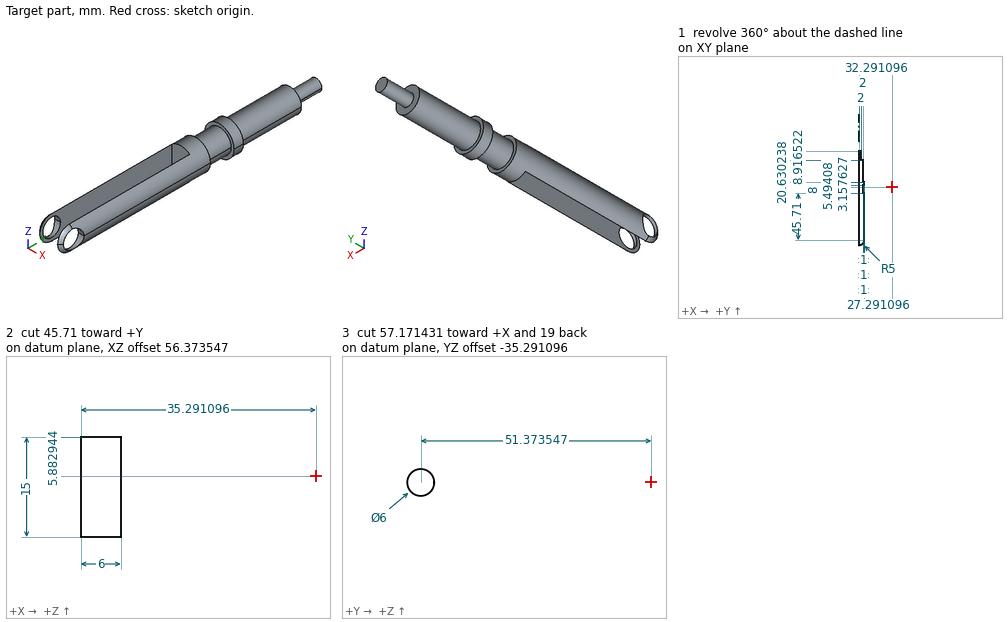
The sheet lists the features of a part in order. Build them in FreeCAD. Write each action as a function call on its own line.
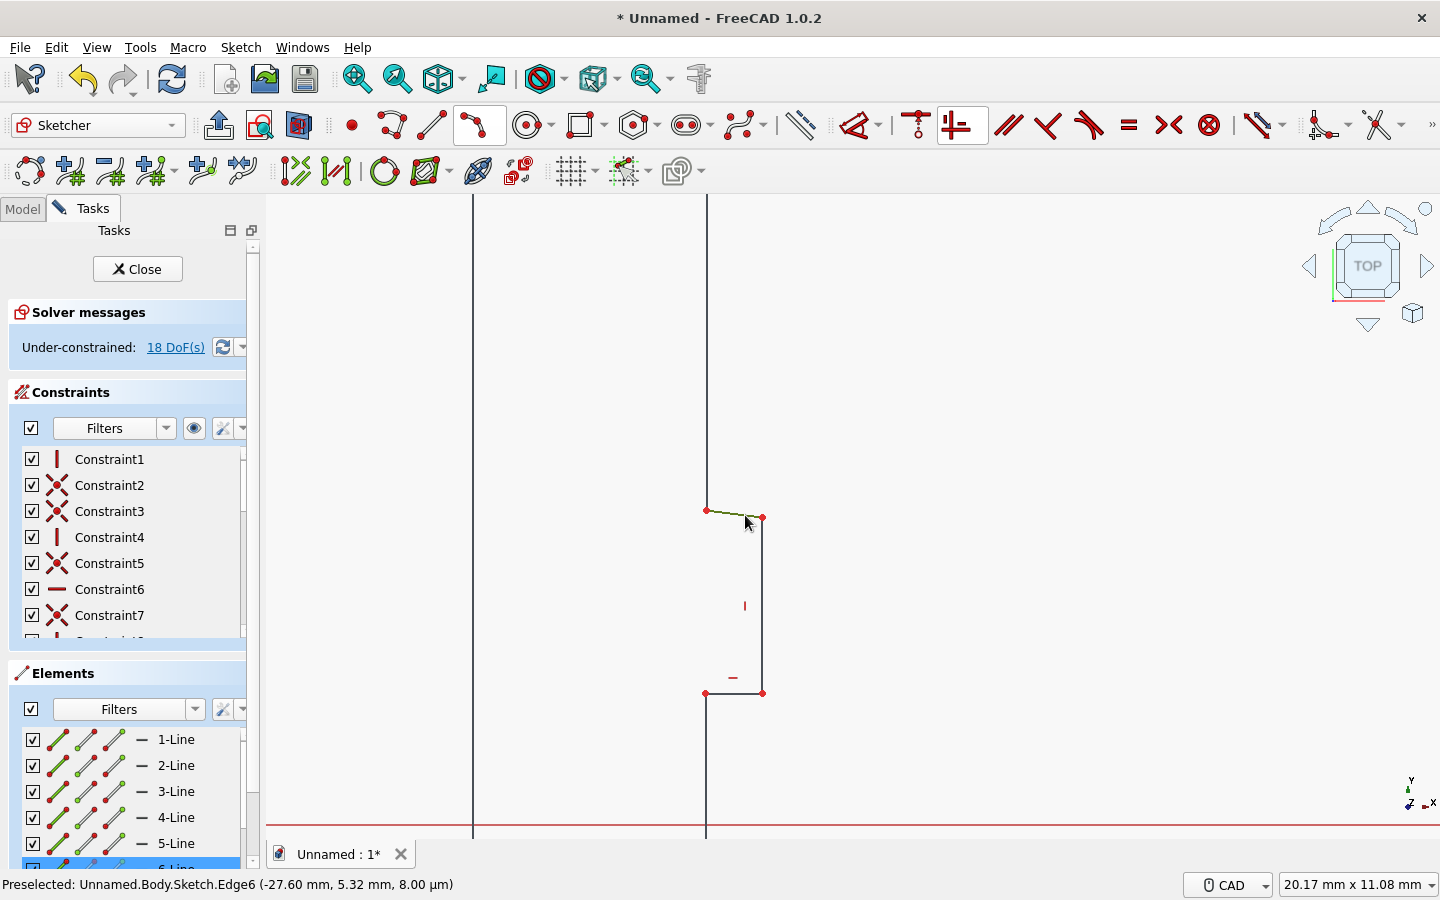
click(982, 126)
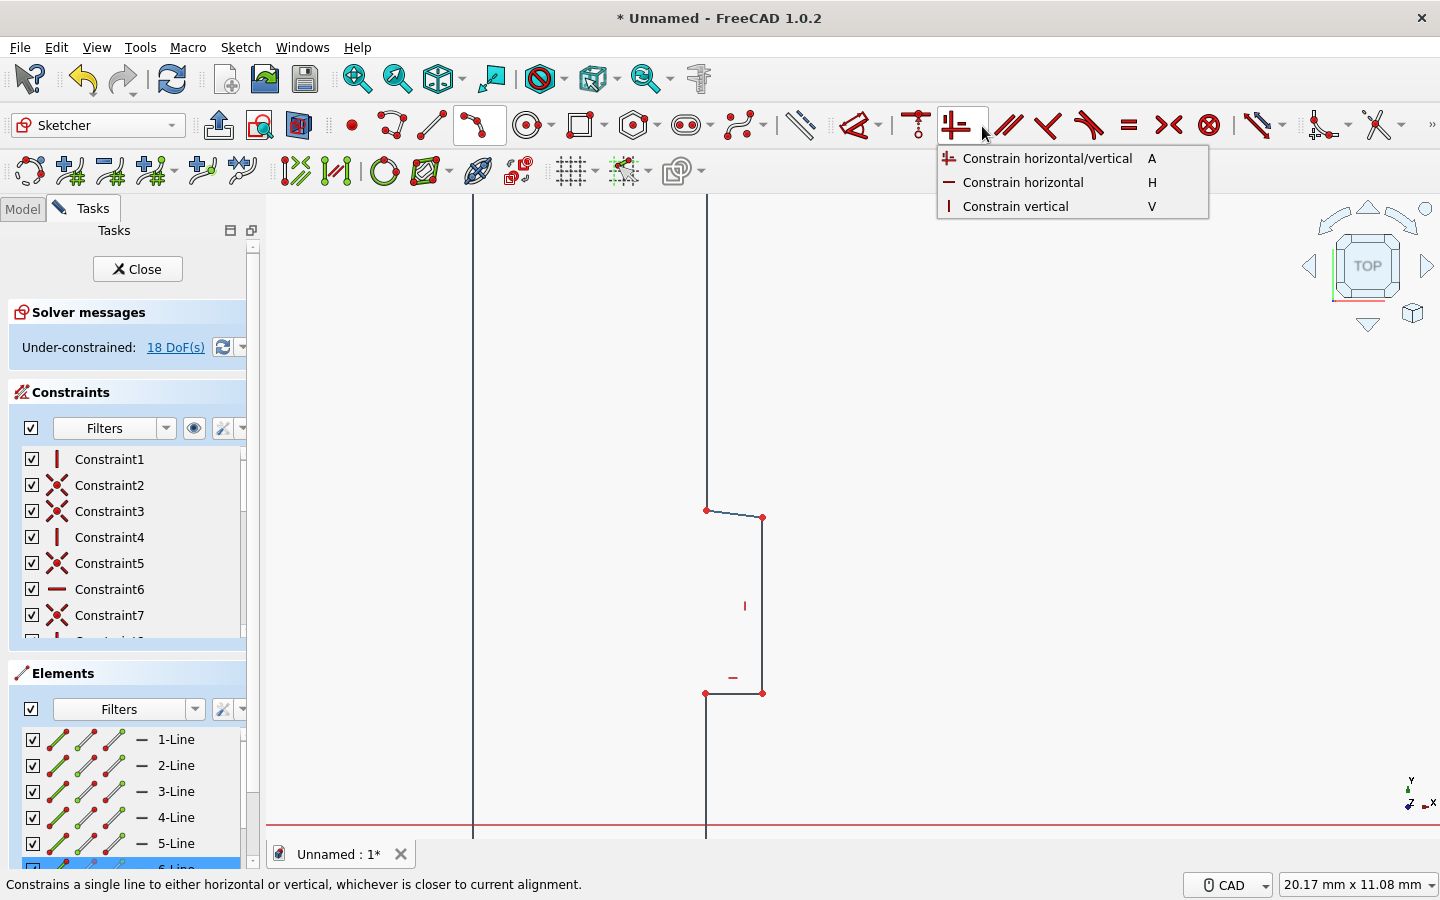
click(1073, 182)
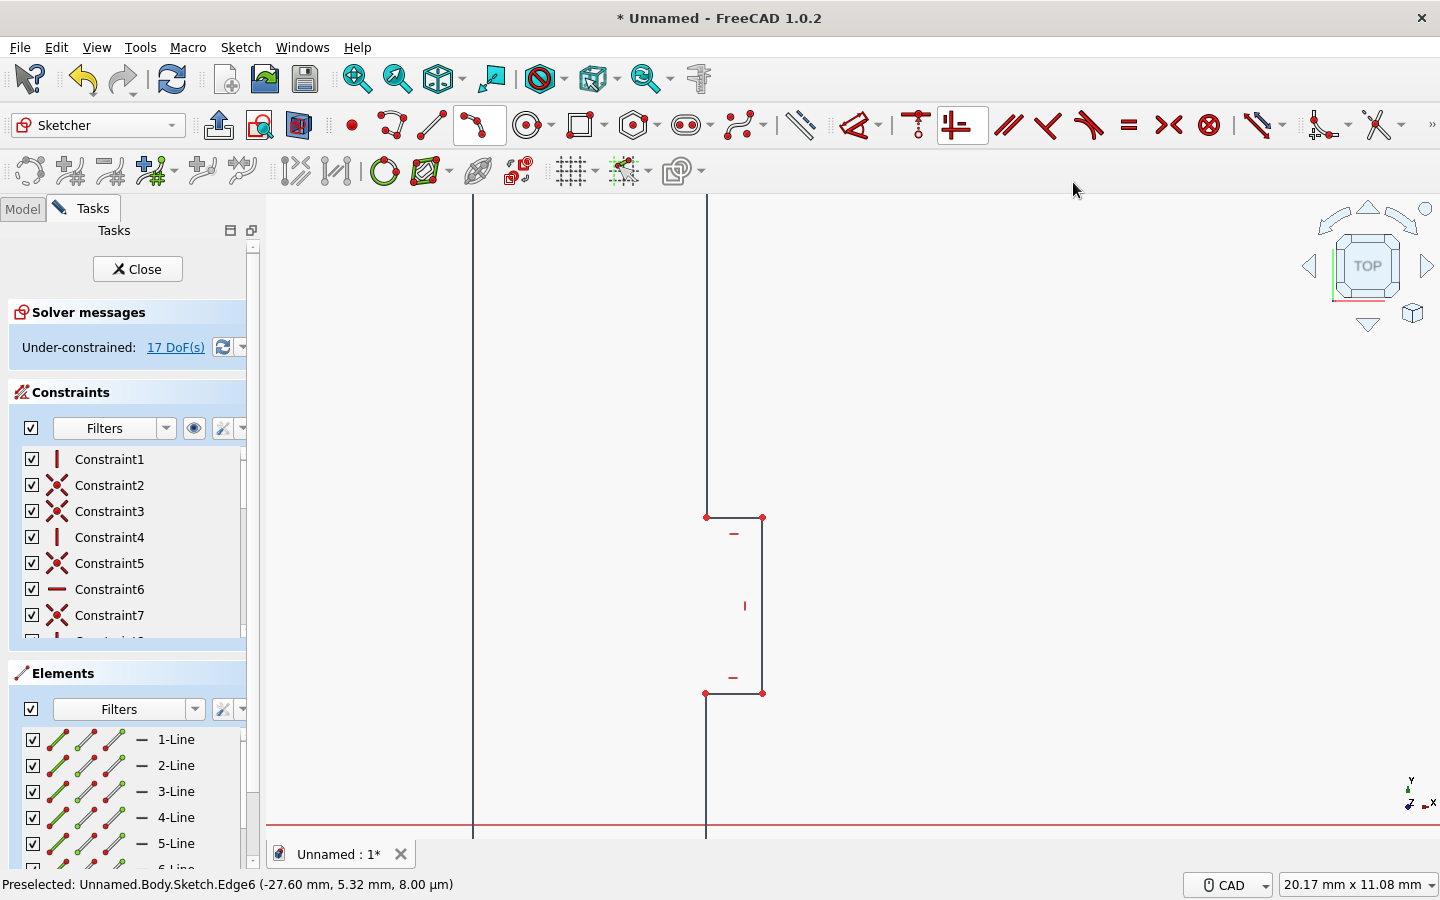
scroll(744, 525, down, 14)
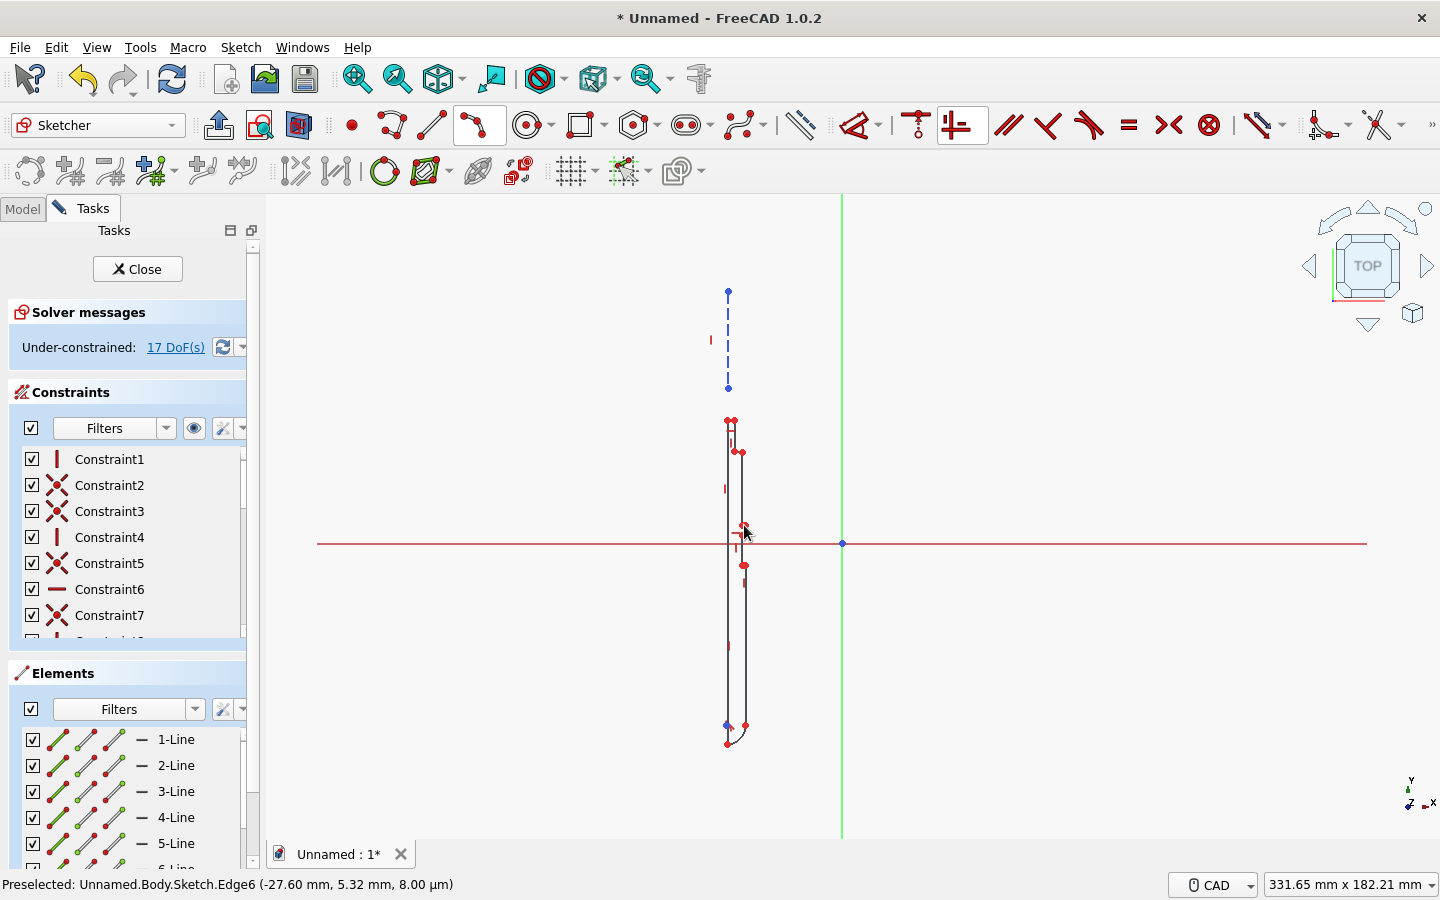
scroll(740, 452, up, 10)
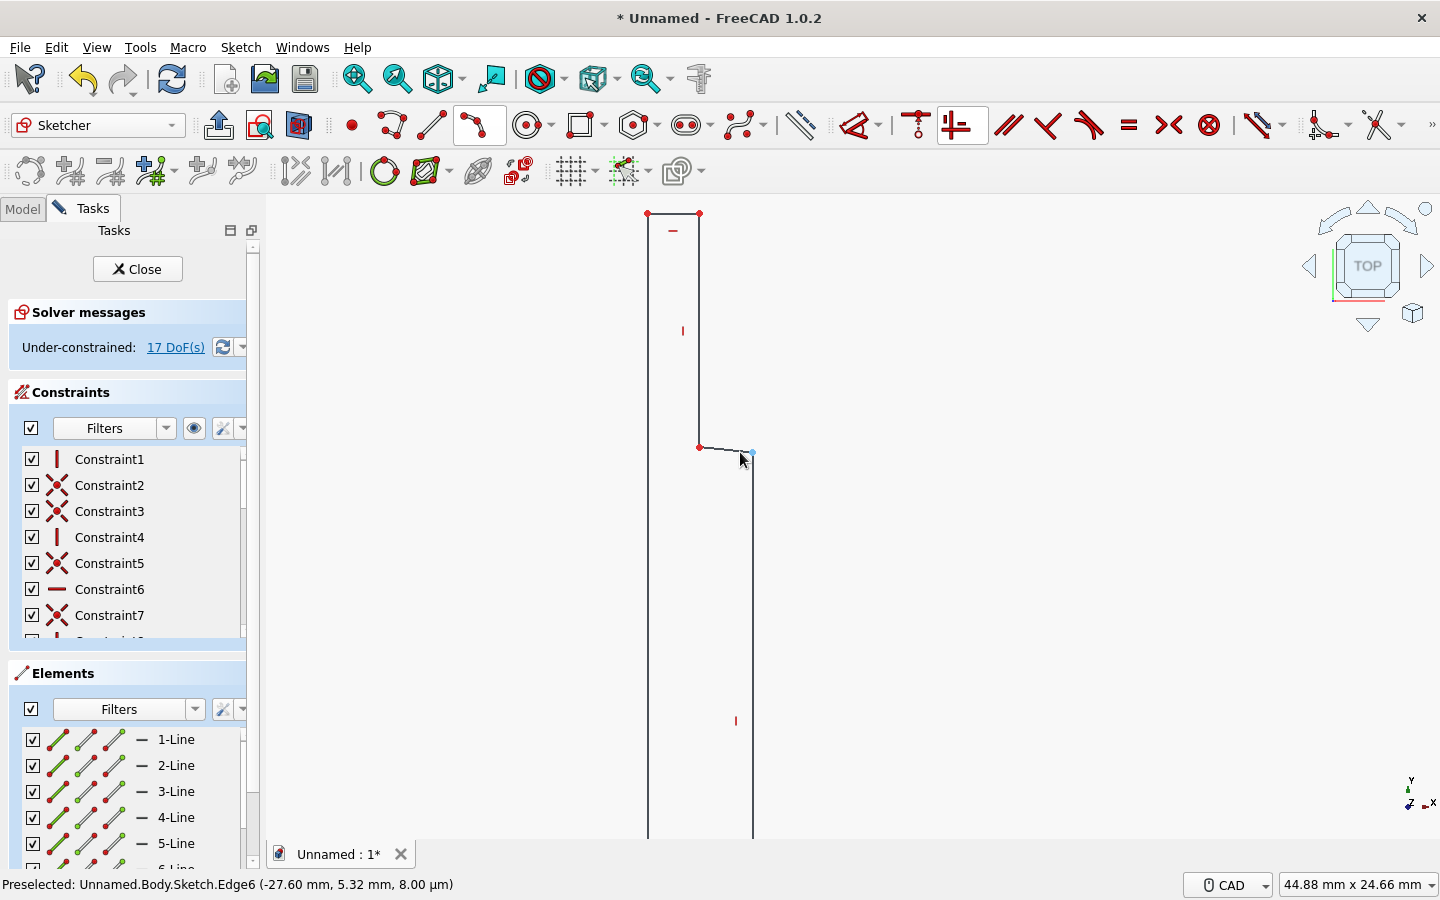
click(737, 451)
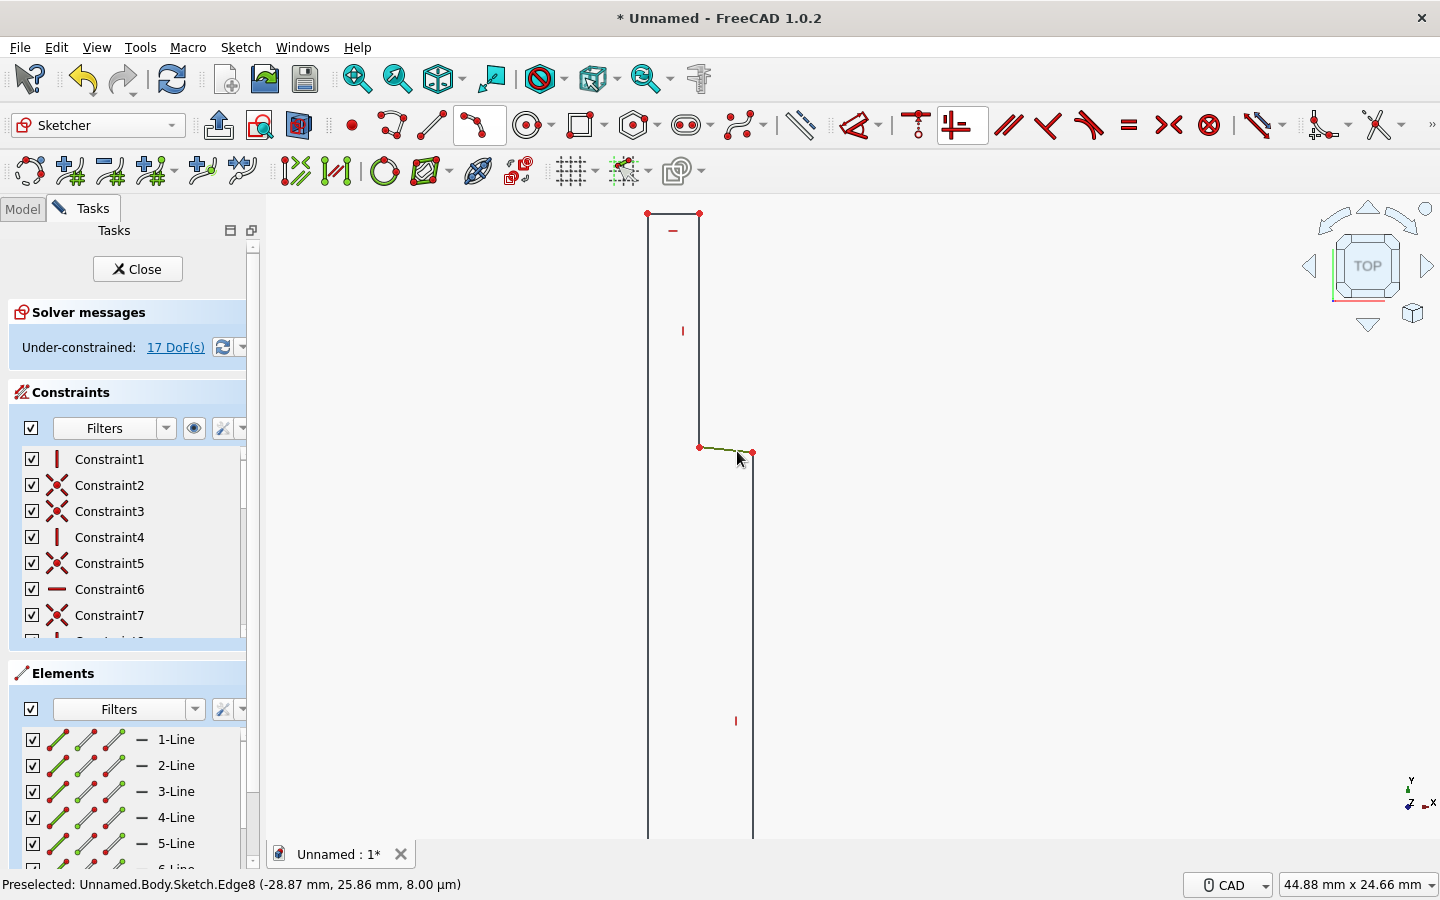
key(h)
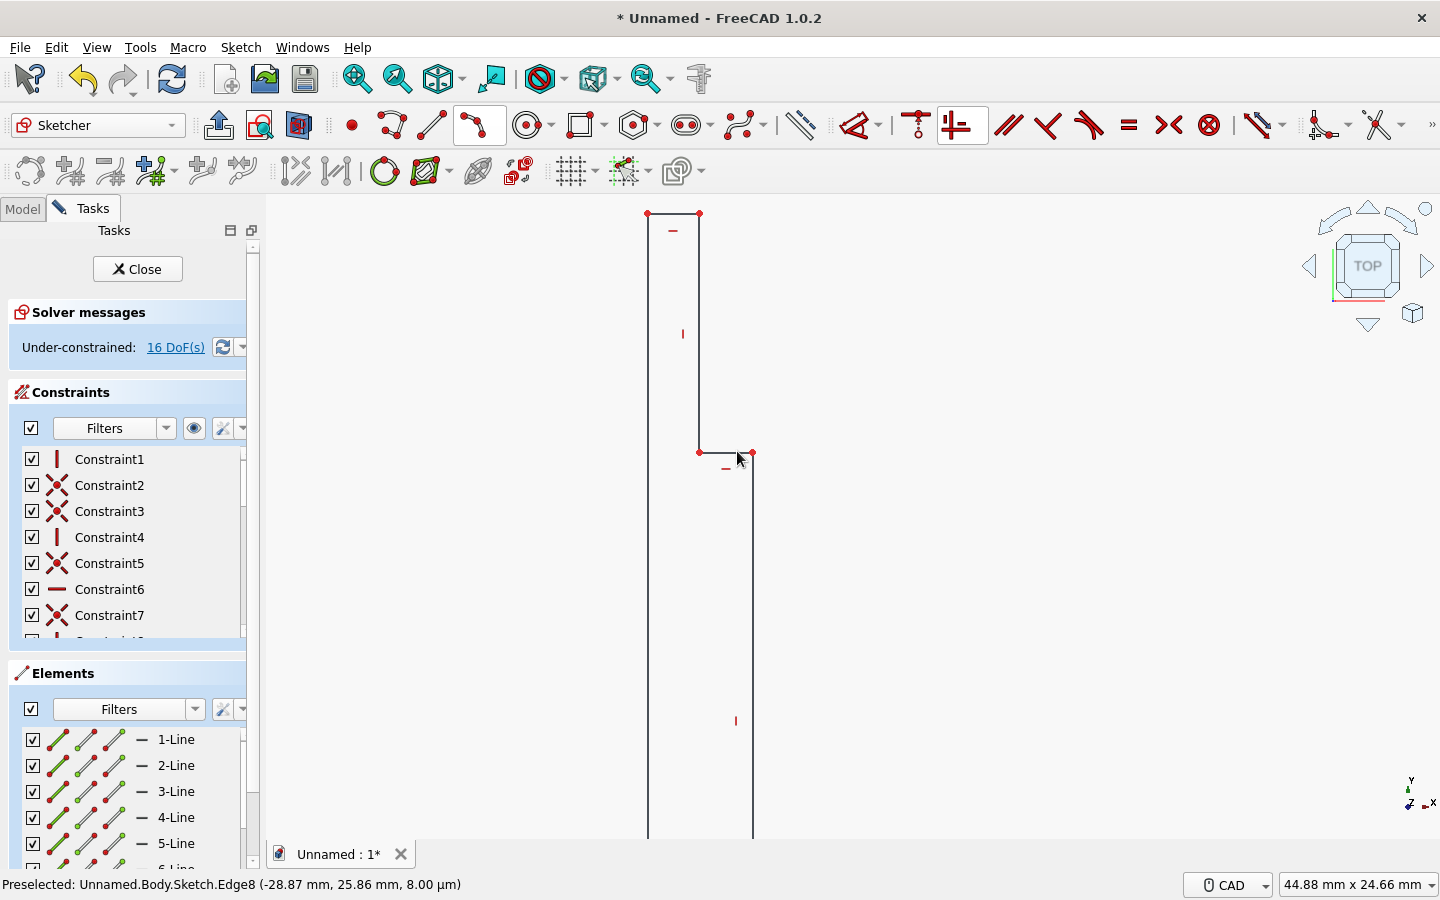
scroll(740, 452, down, 10)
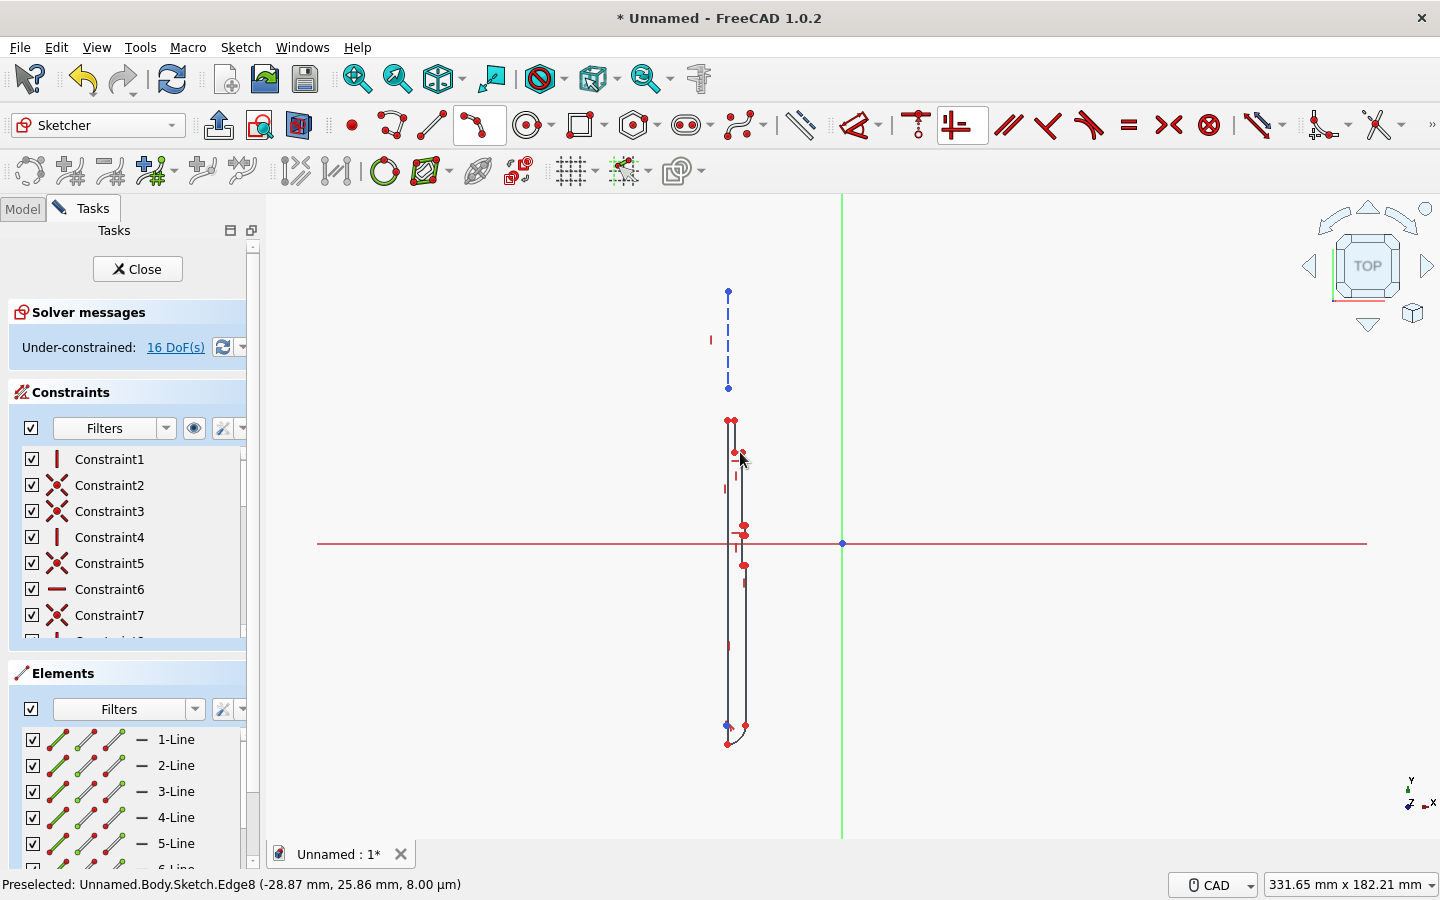
scroll(736, 742, up, 5)